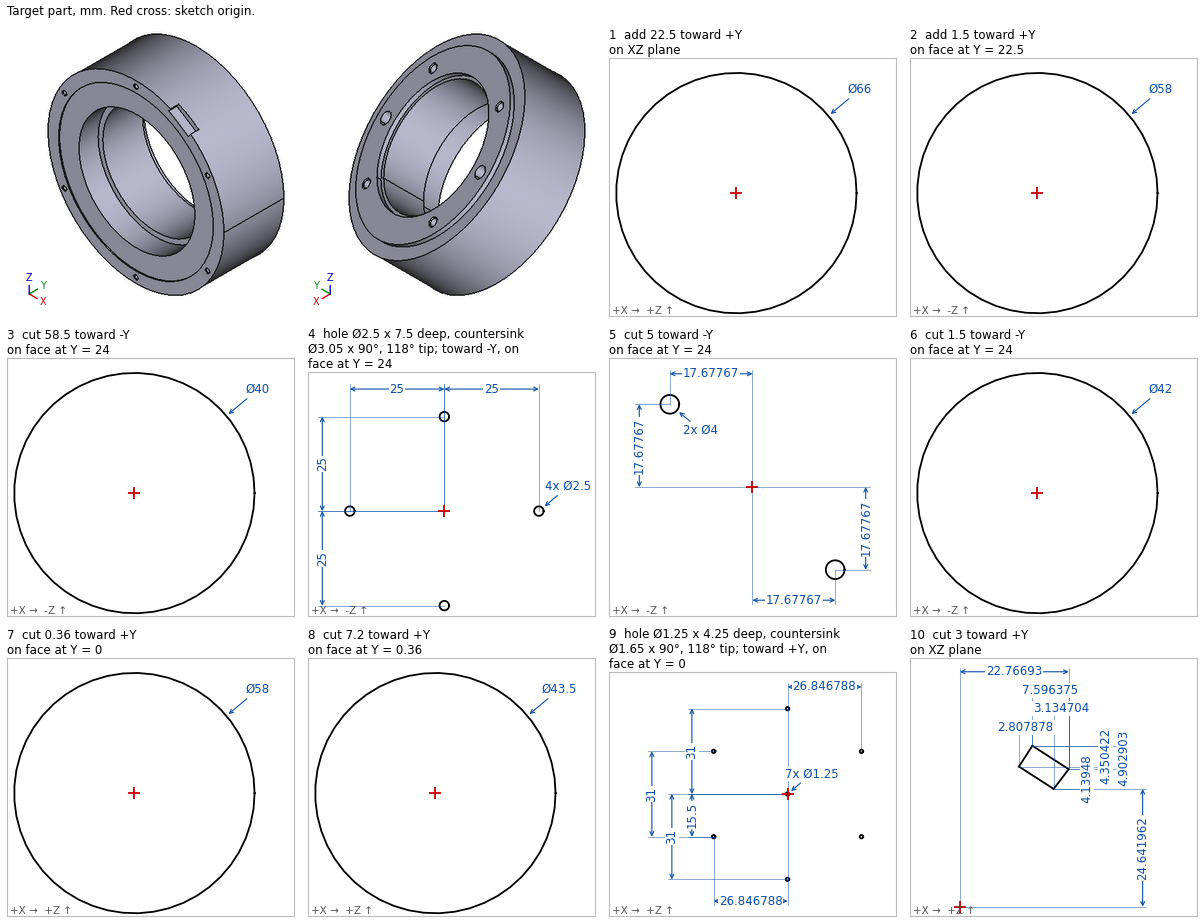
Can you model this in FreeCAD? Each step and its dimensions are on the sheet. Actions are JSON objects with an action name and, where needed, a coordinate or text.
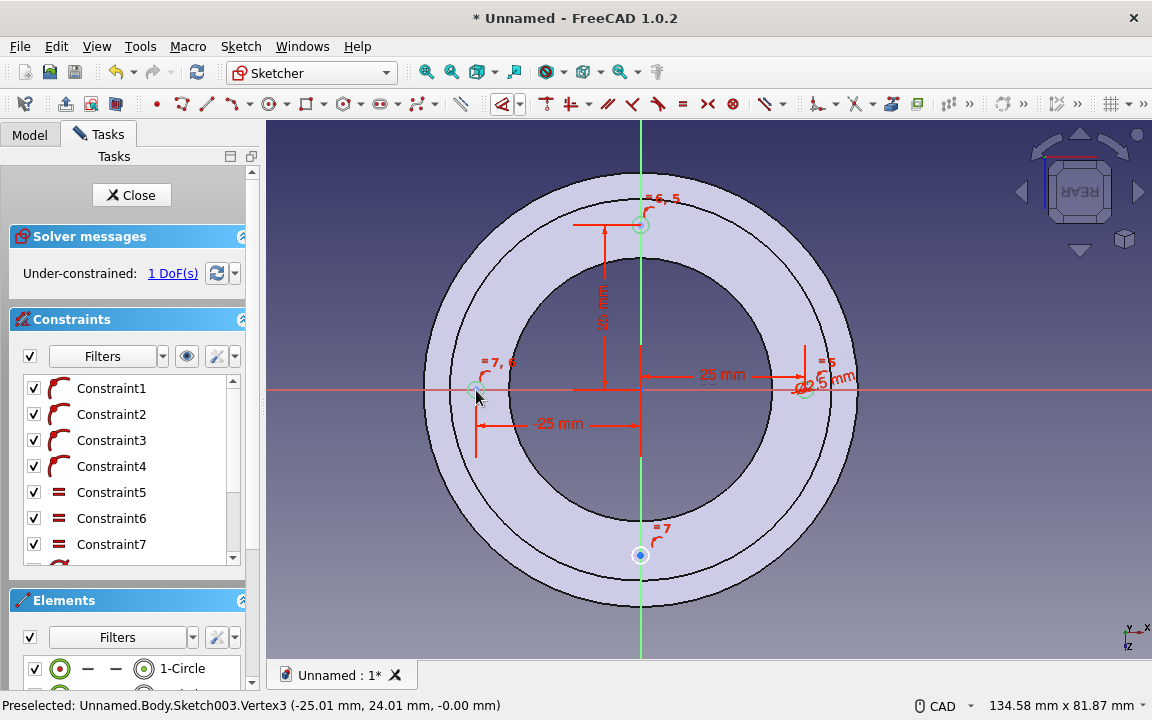
{"action": "left_click", "coordinate": [641, 555]}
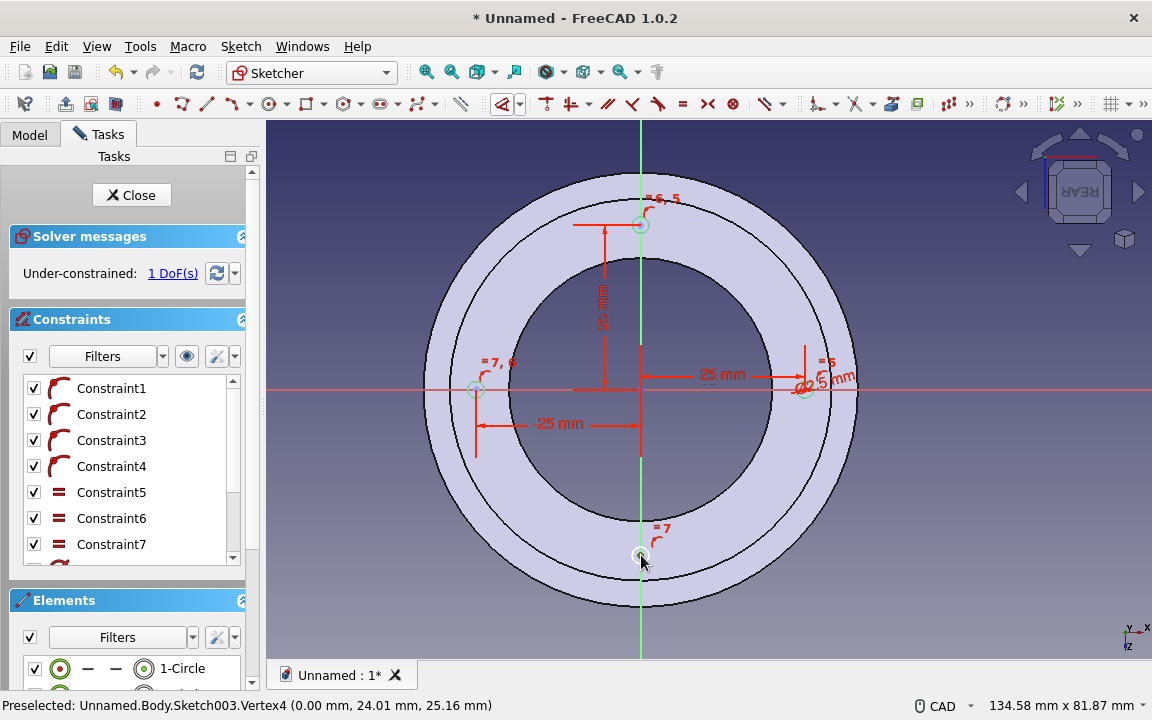
{"action": "left_click", "coordinate": [520, 104]}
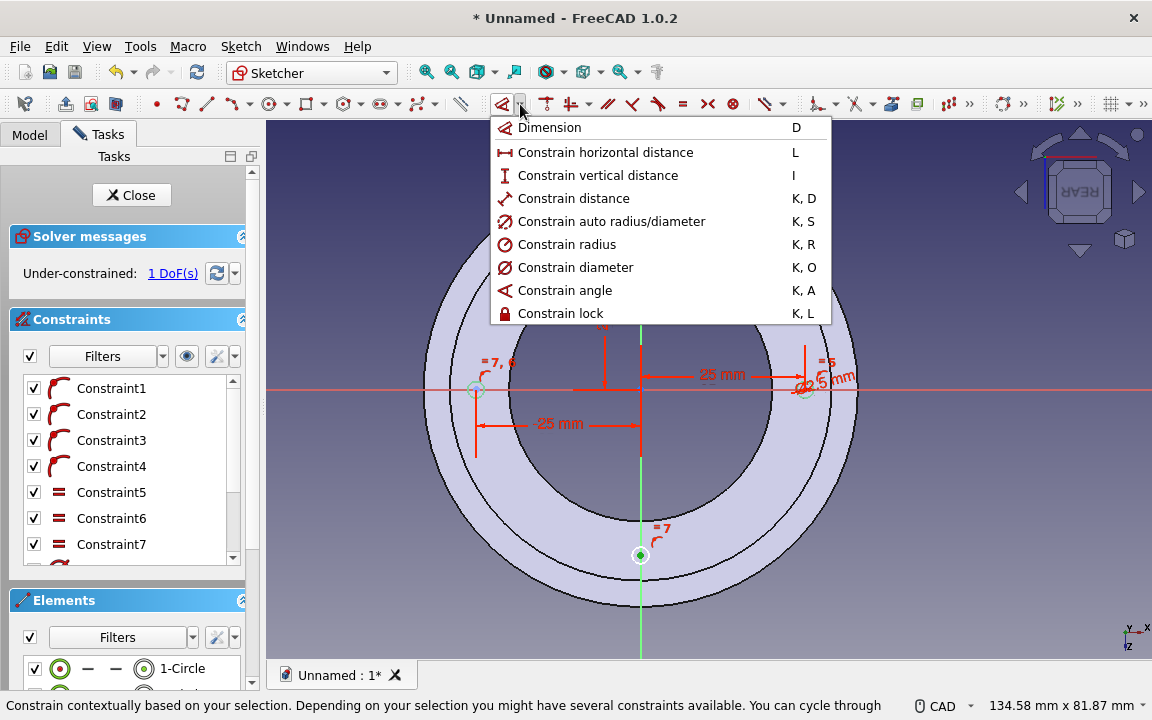
{"action": "left_click", "coordinate": [661, 176]}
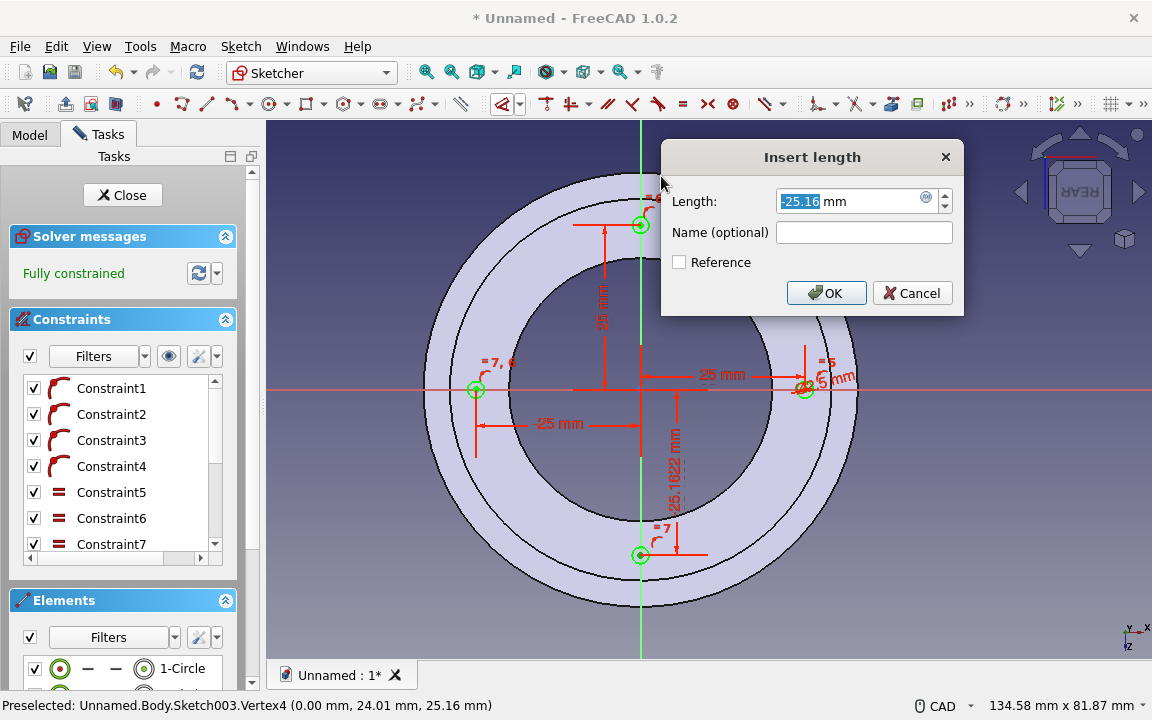
{"action": "type", "text": "-25"}
{"action": "key", "text": "Return"}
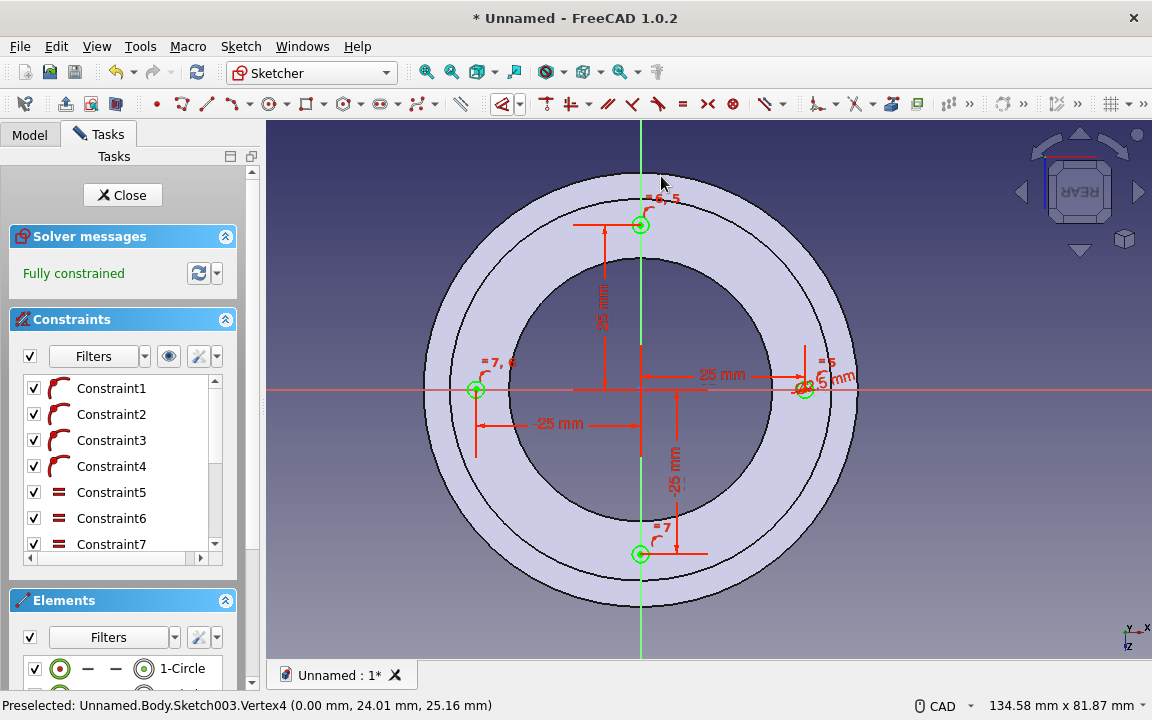
{"action": "left_click", "coordinate": [123, 195]}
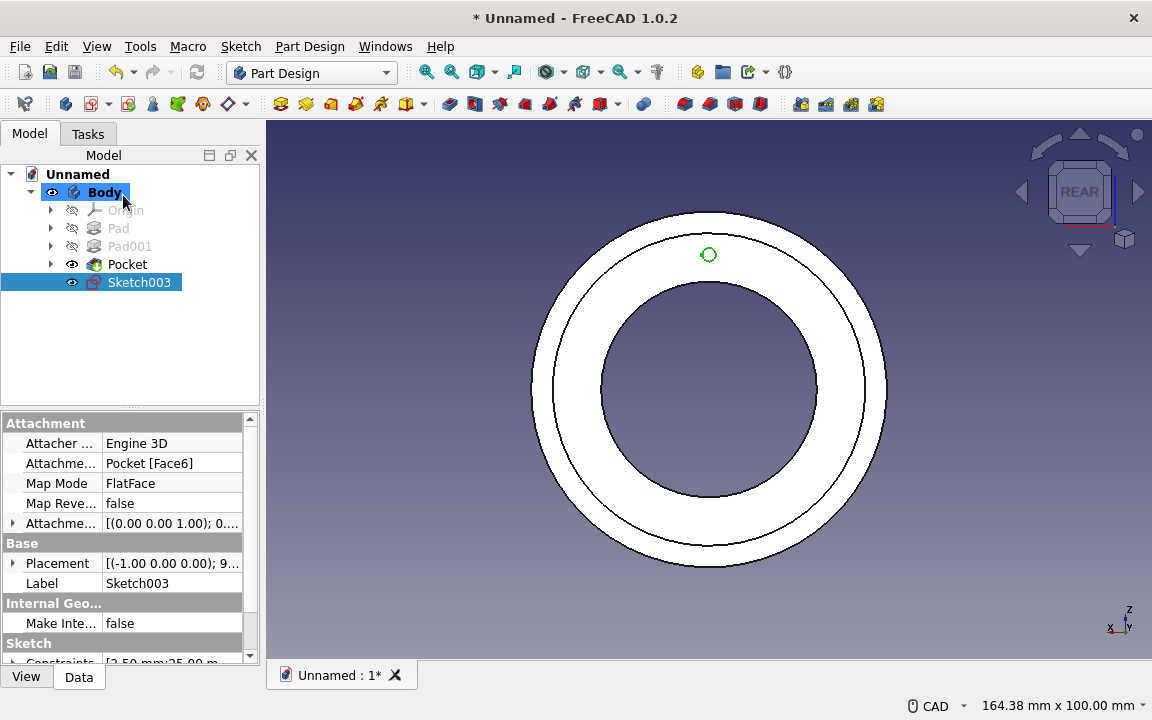
{"action": "left_click", "coordinate": [475, 104]}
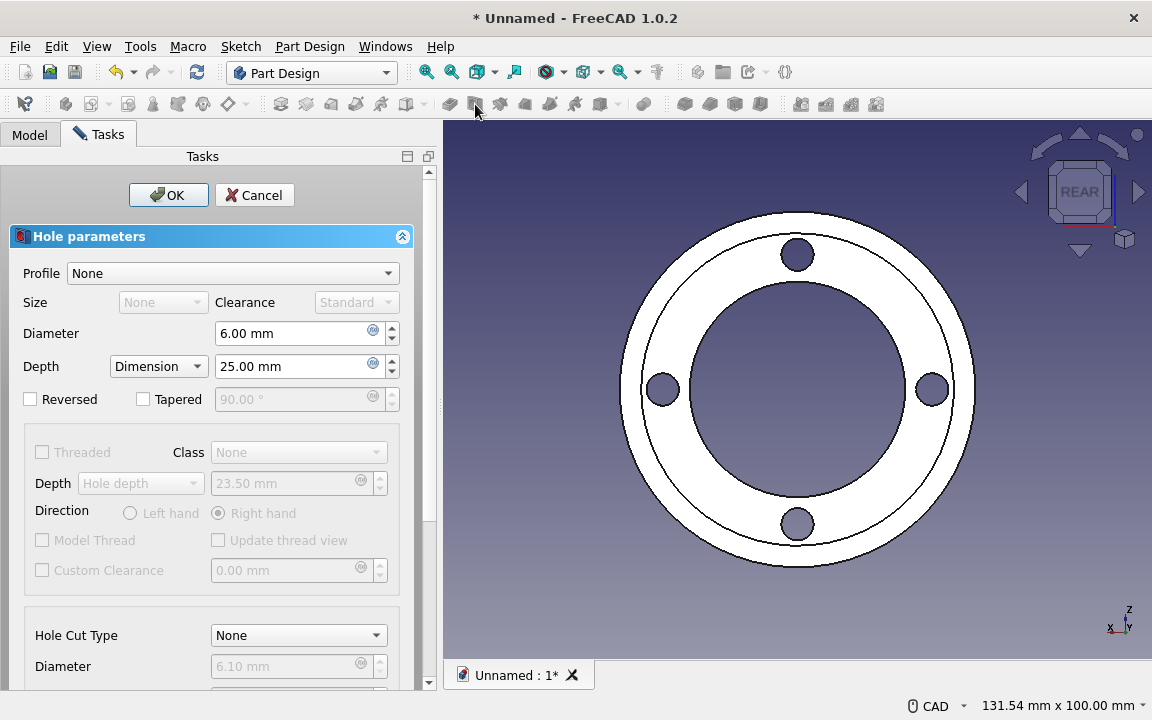
{"action": "triple_click", "coordinate": [300, 334]}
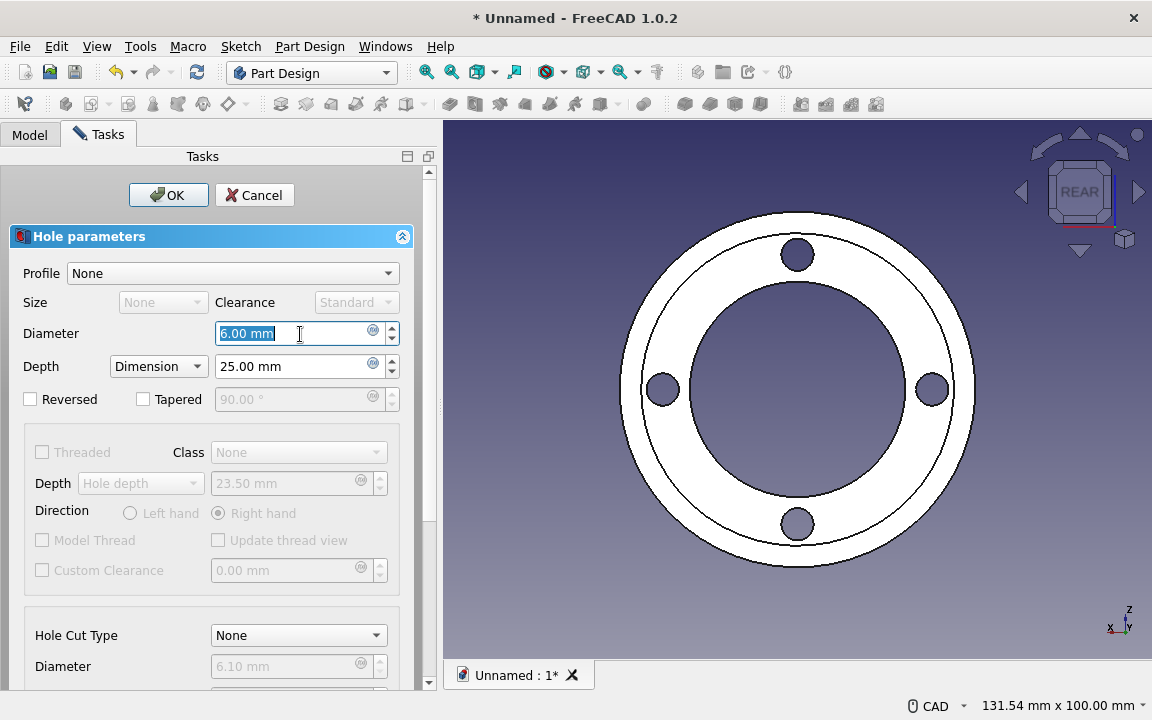
{"action": "type", "text": "2.5"}
{"action": "key", "text": "Tab"}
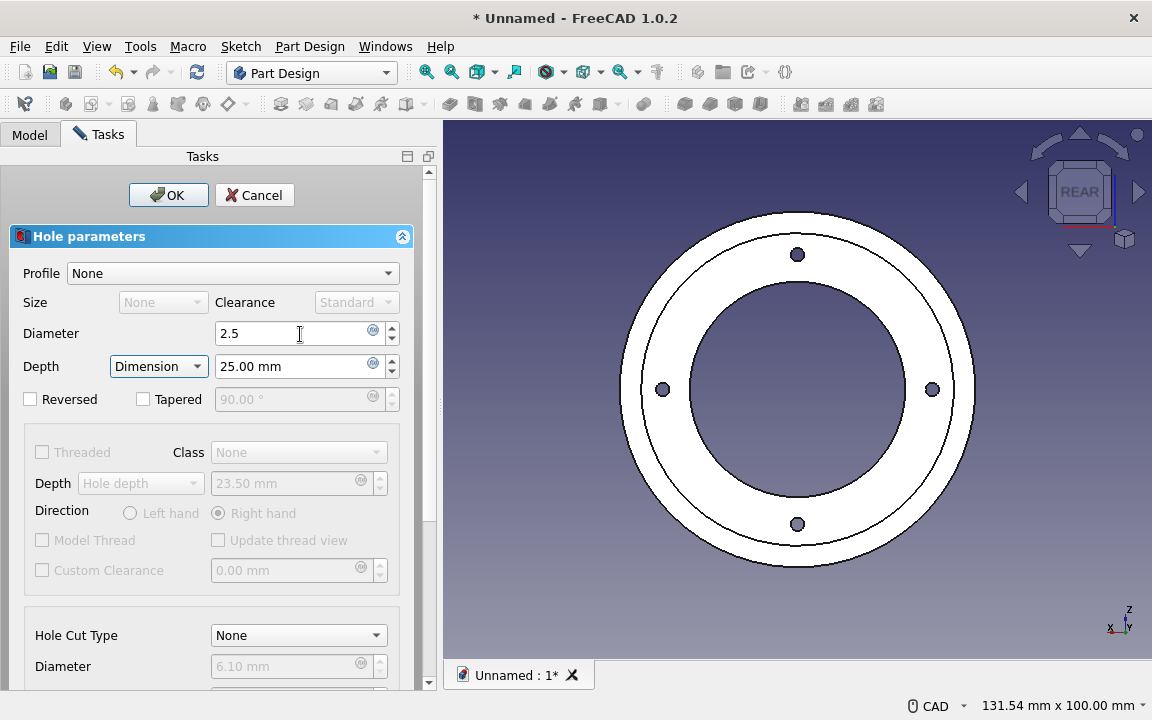
{"action": "triple_click", "coordinate": [300, 366]}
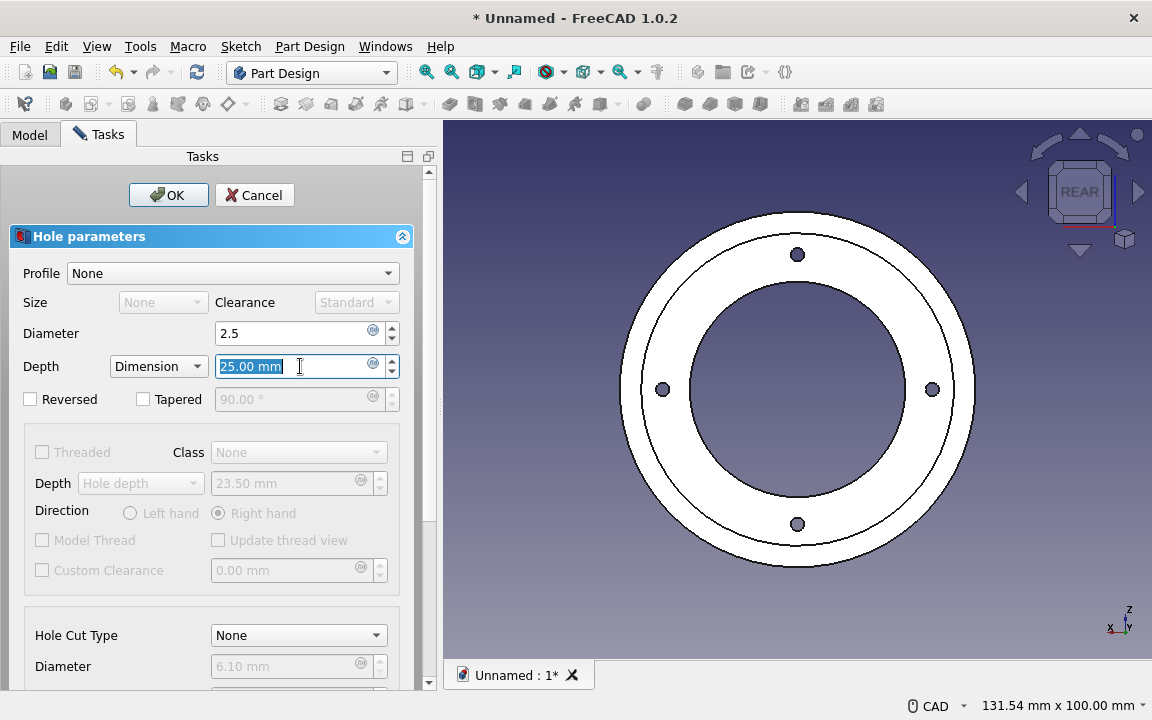
{"action": "type", "text": "7.5"}
{"action": "key", "text": "Tab"}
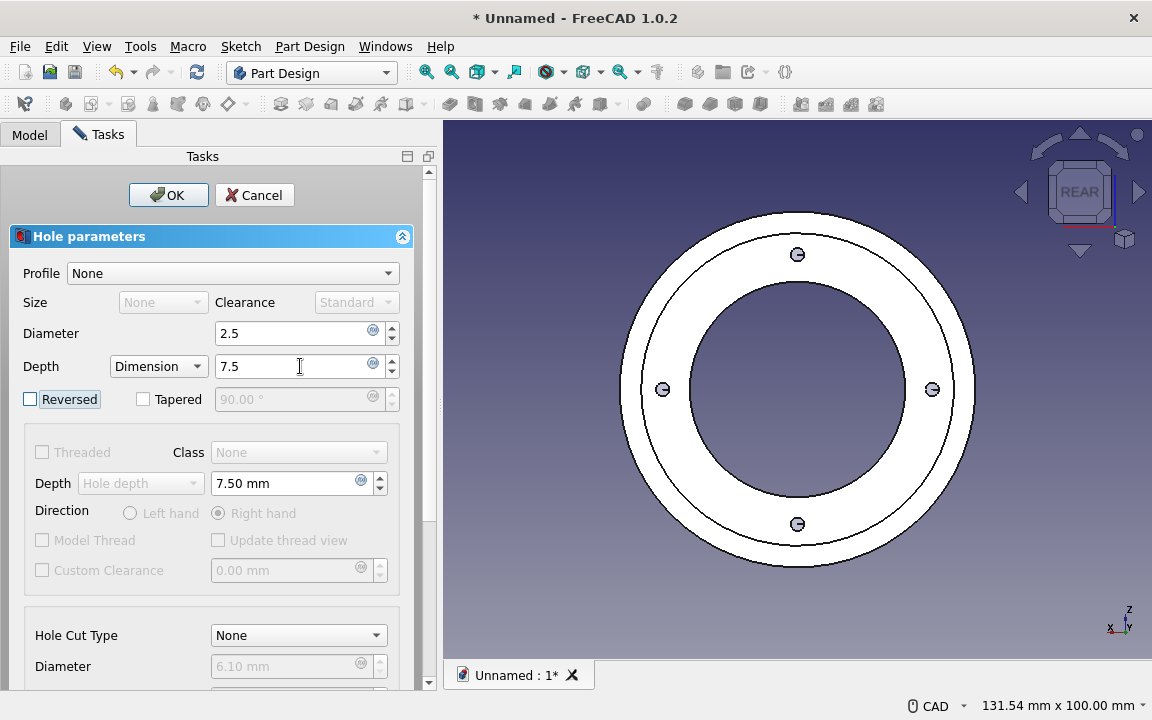
{"action": "left_click", "coordinate": [300, 636]}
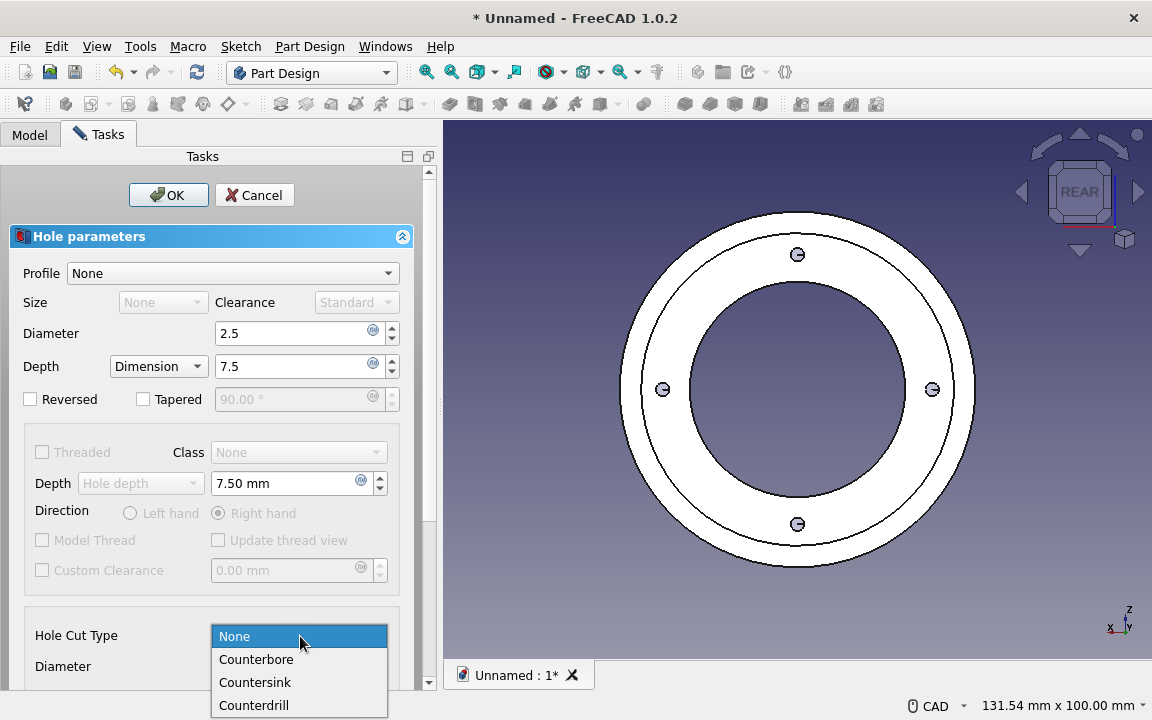
{"action": "left_click", "coordinate": [298, 682]}